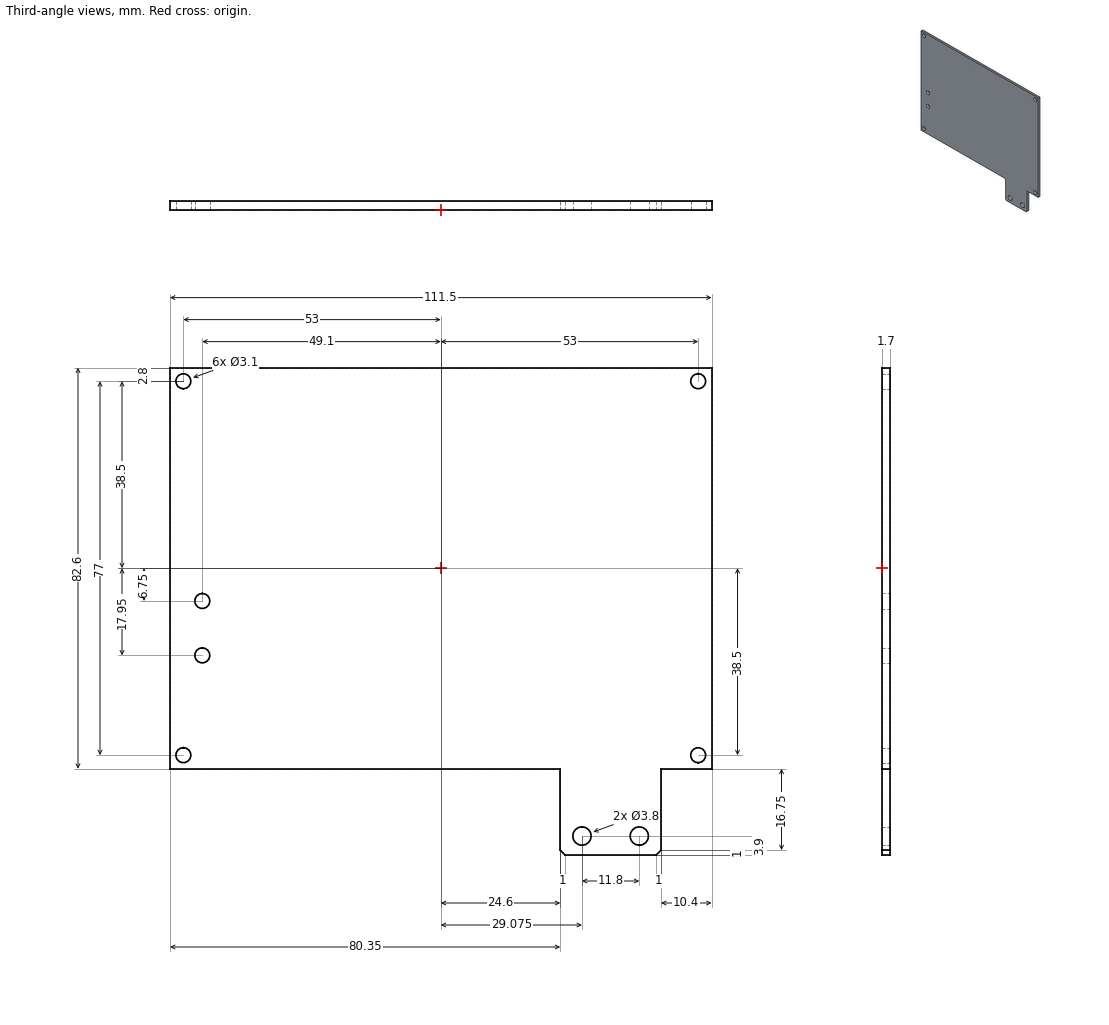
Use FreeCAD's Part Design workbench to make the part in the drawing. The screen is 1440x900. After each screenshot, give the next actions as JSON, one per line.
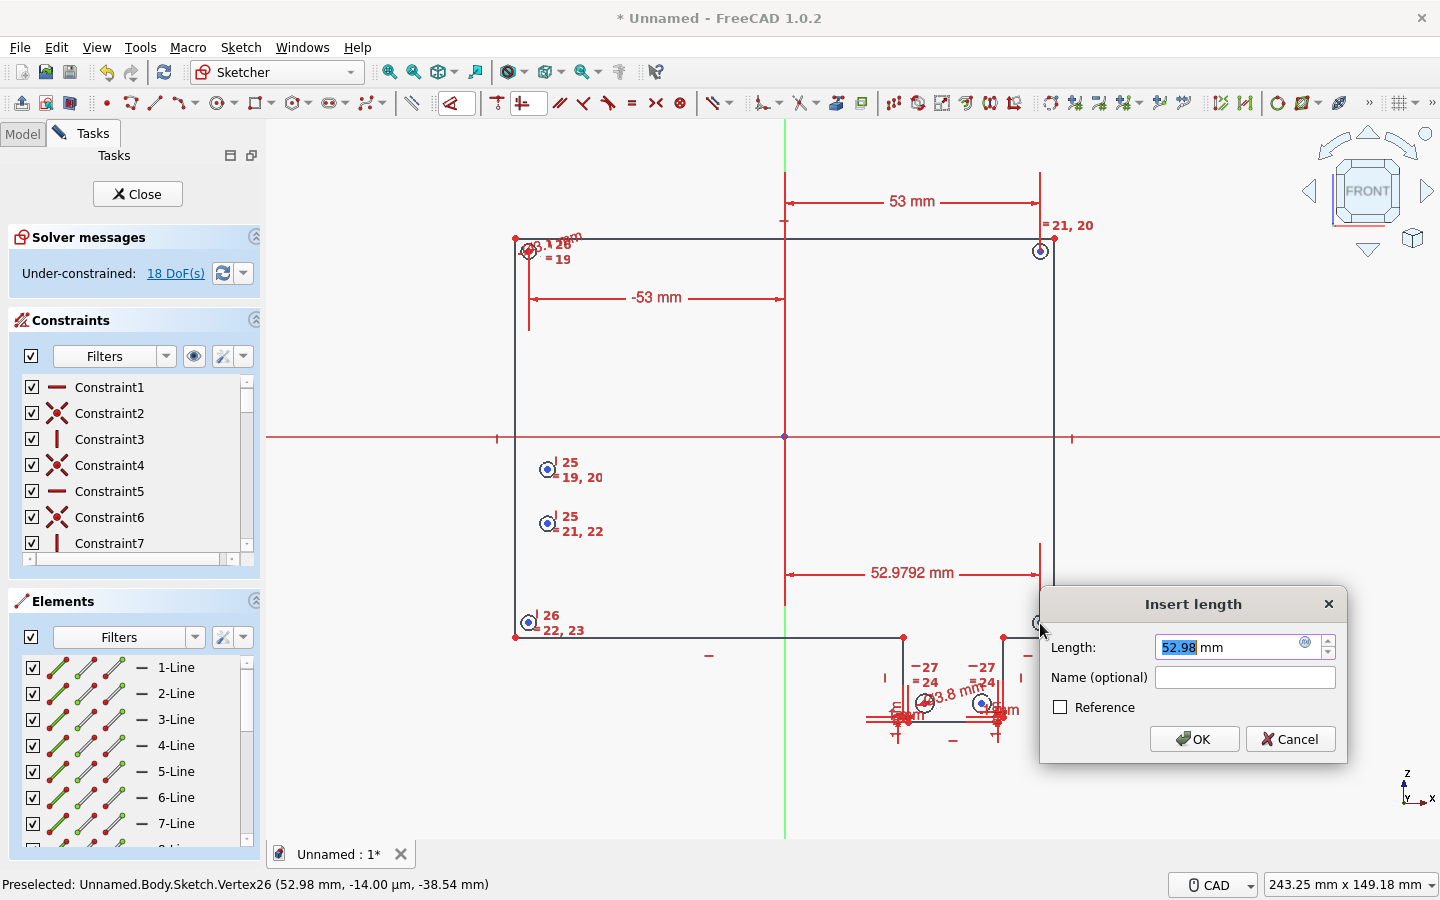
{"action": "type", "text": "53"}
{"action": "key", "text": "Return"}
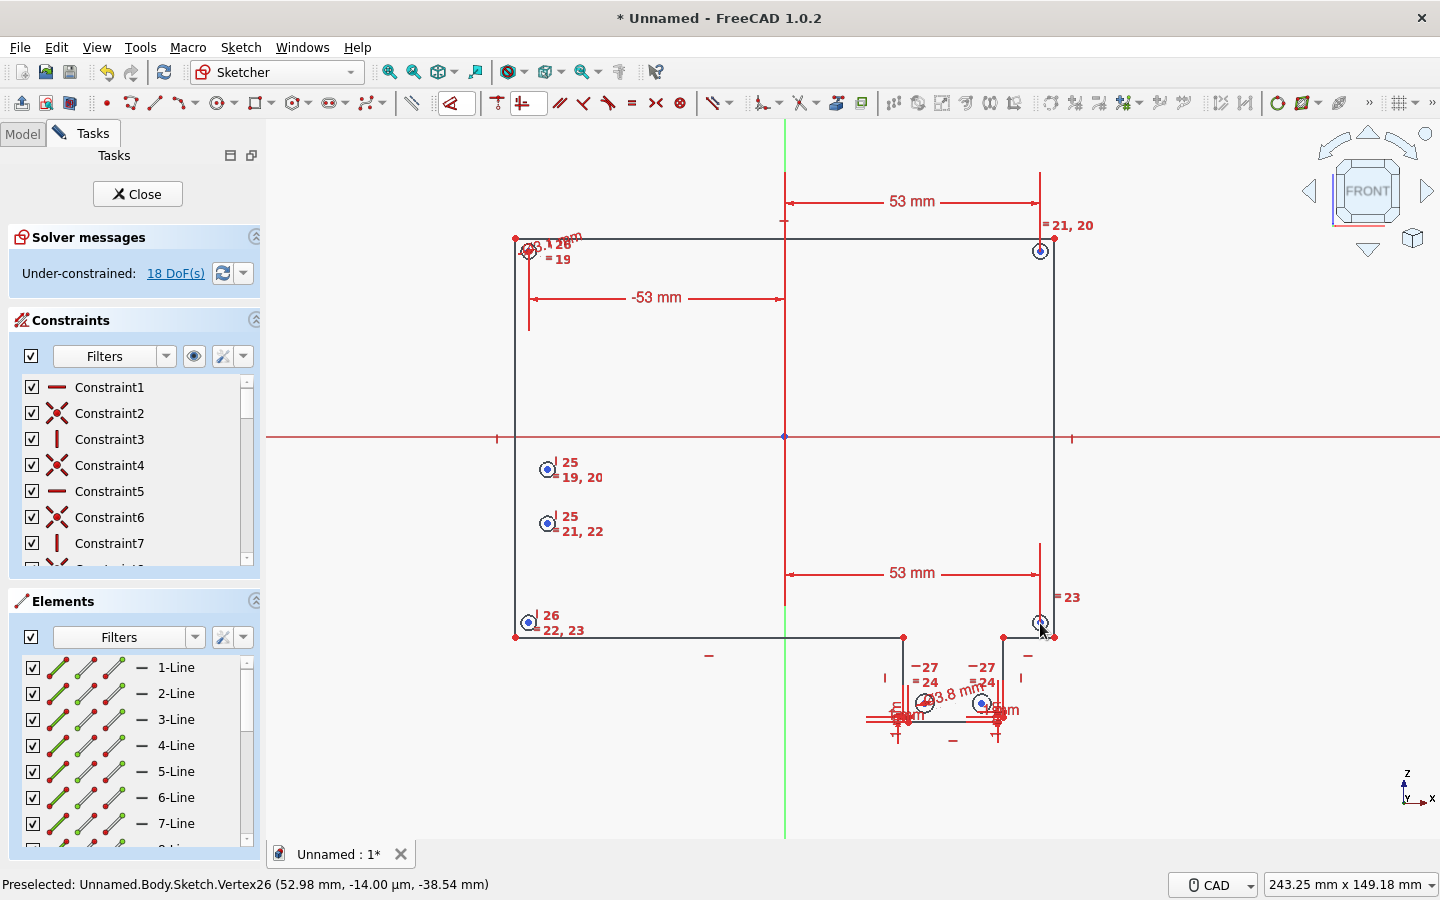
{"action": "left_click", "coordinate": [529, 251]}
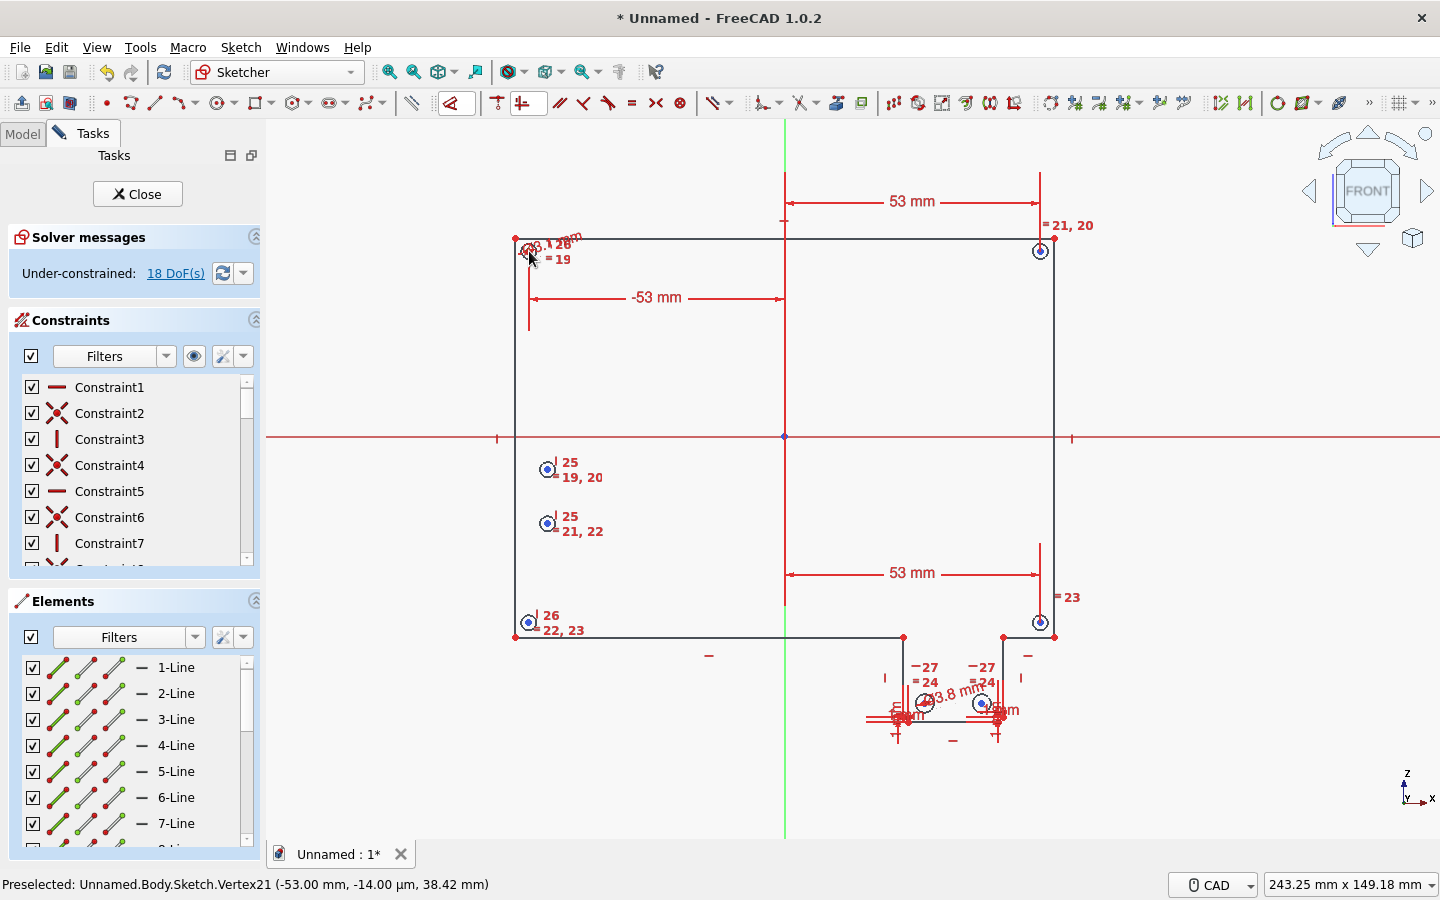
{"action": "left_click", "coordinate": [529, 623]}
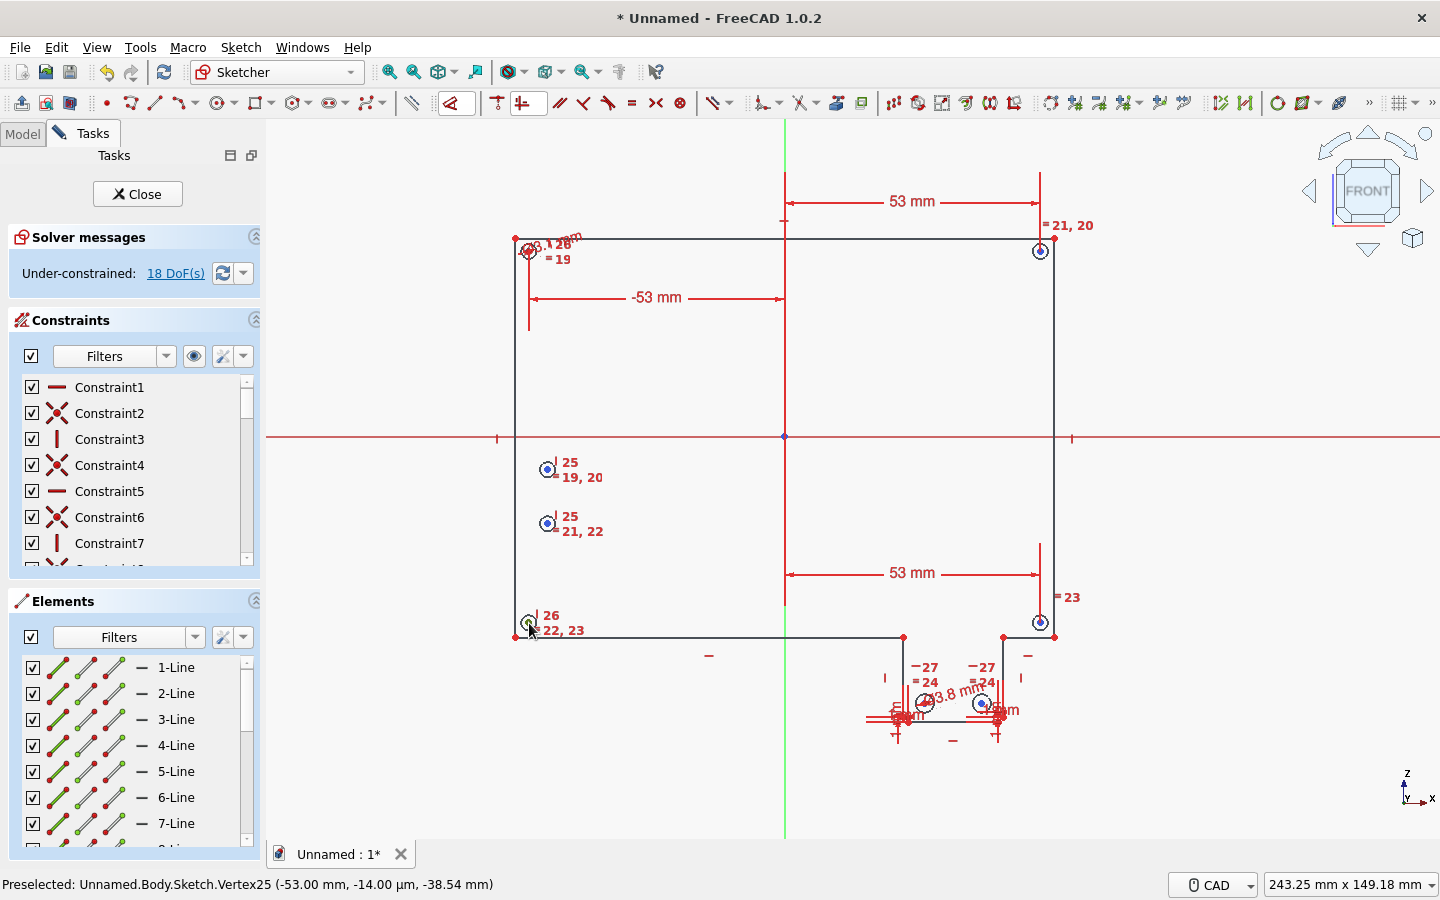
{"action": "left_click", "coordinate": [470, 104]}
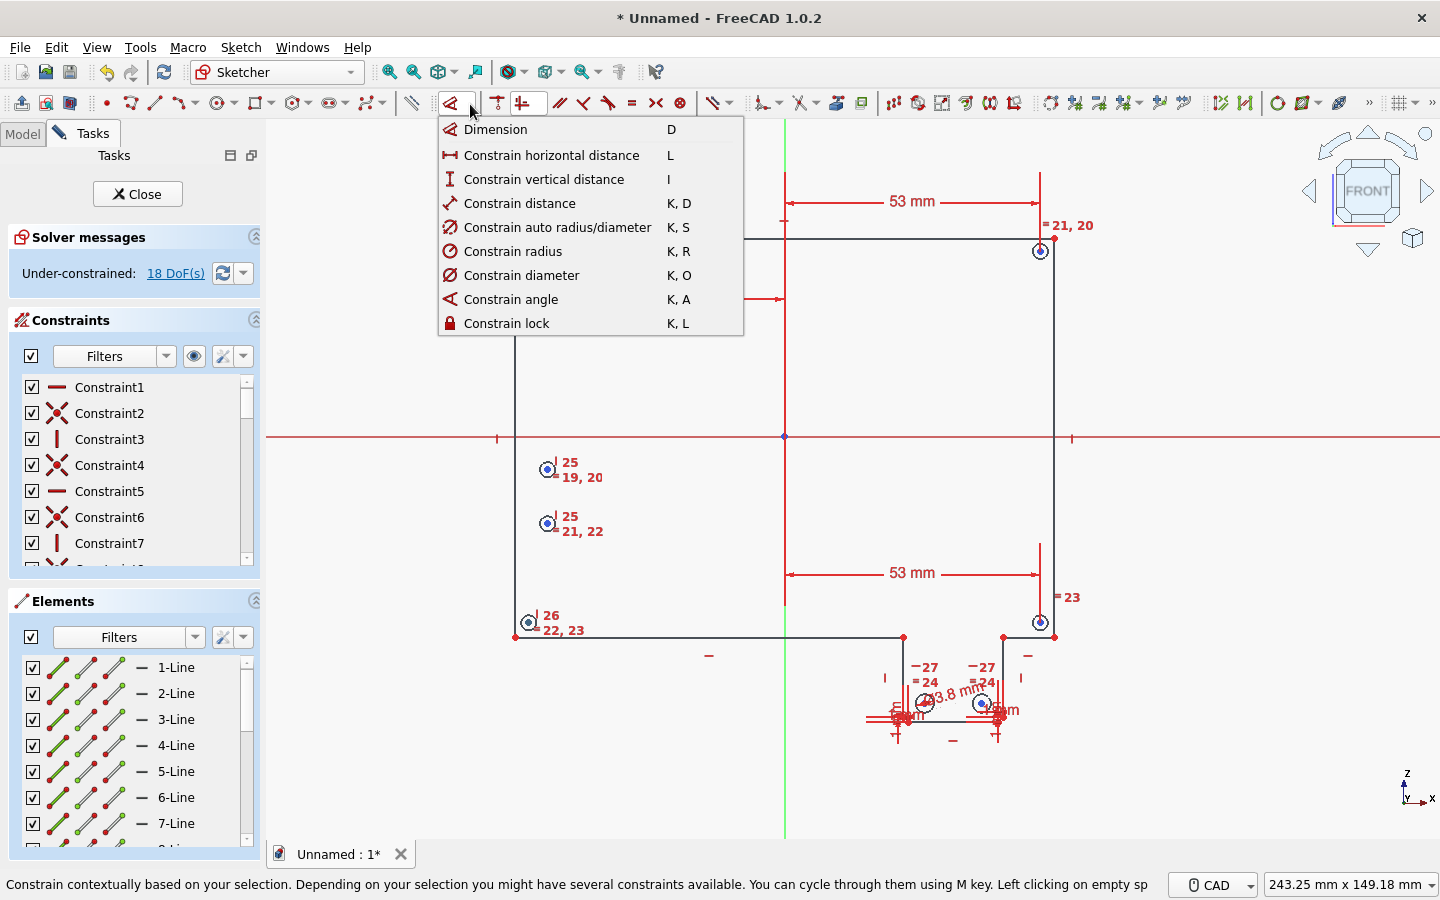
{"action": "left_click", "coordinate": [591, 179]}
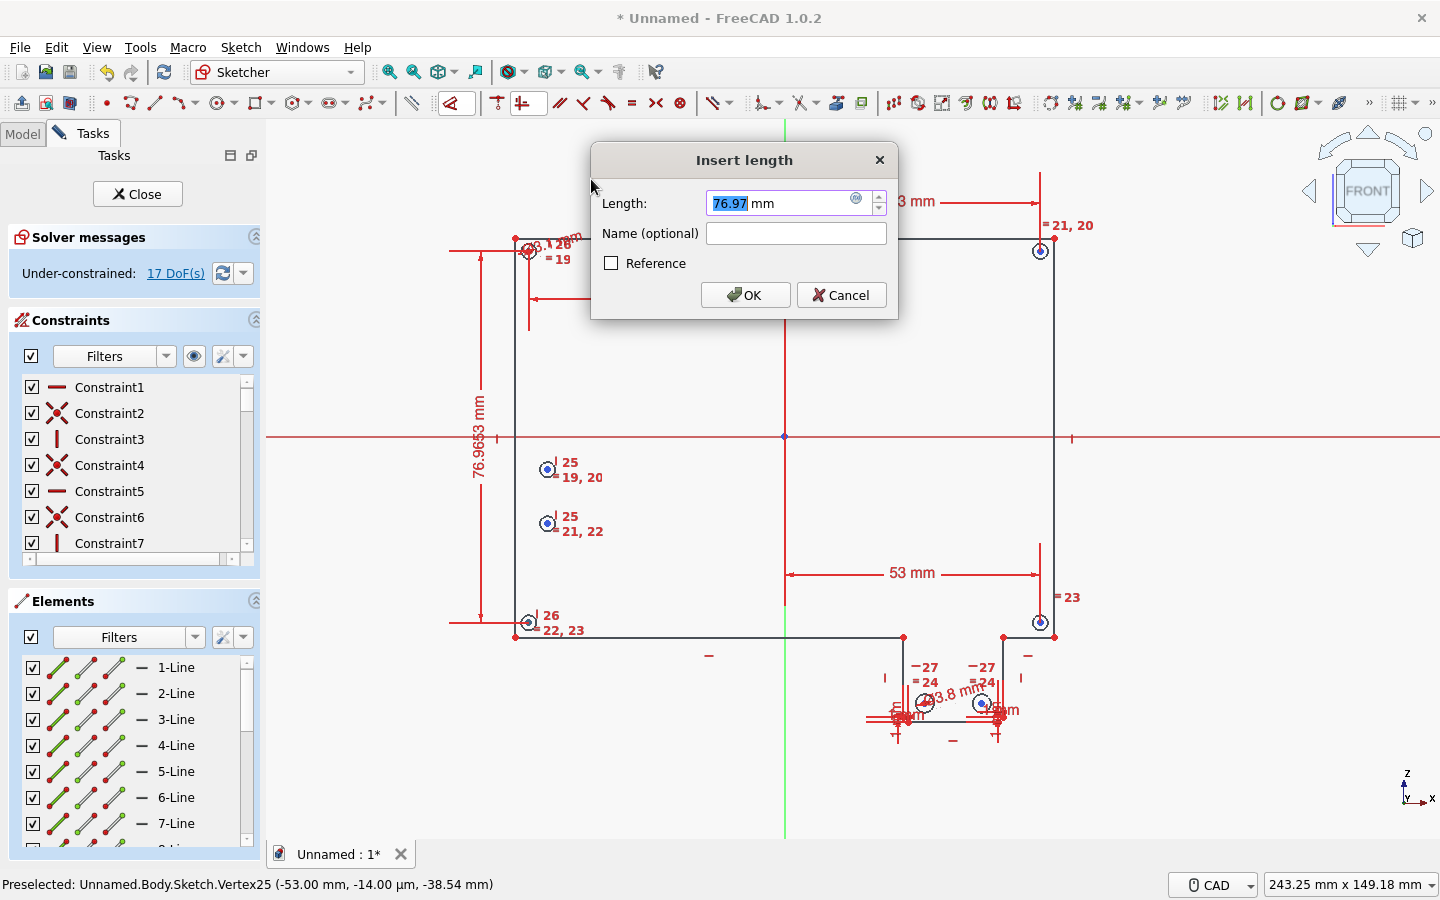
{"action": "type", "text": "77"}
{"action": "key", "text": "Return"}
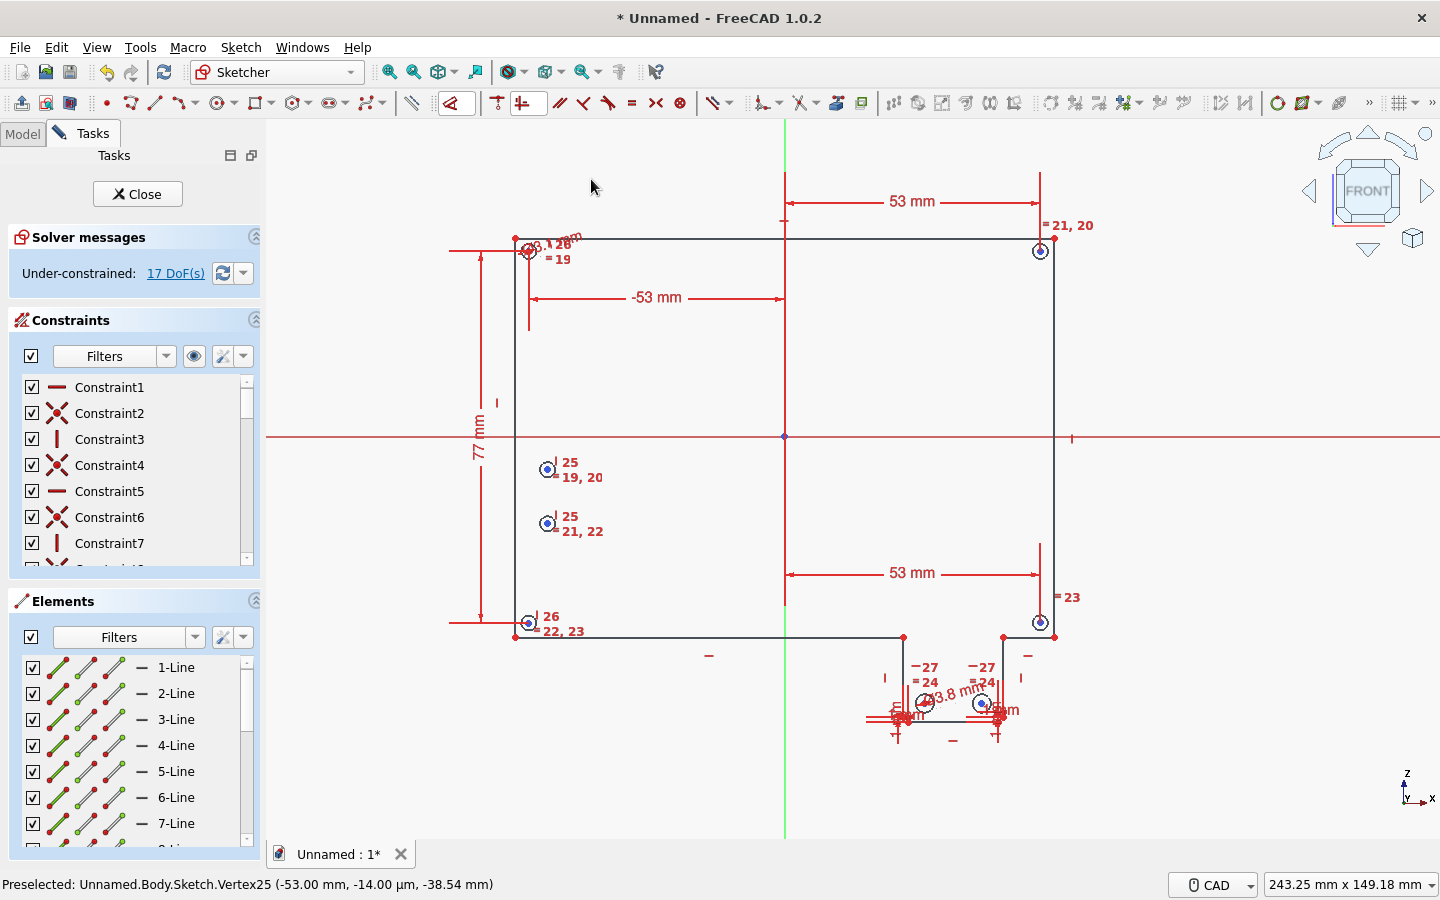
{"action": "left_click", "coordinate": [515, 518]}